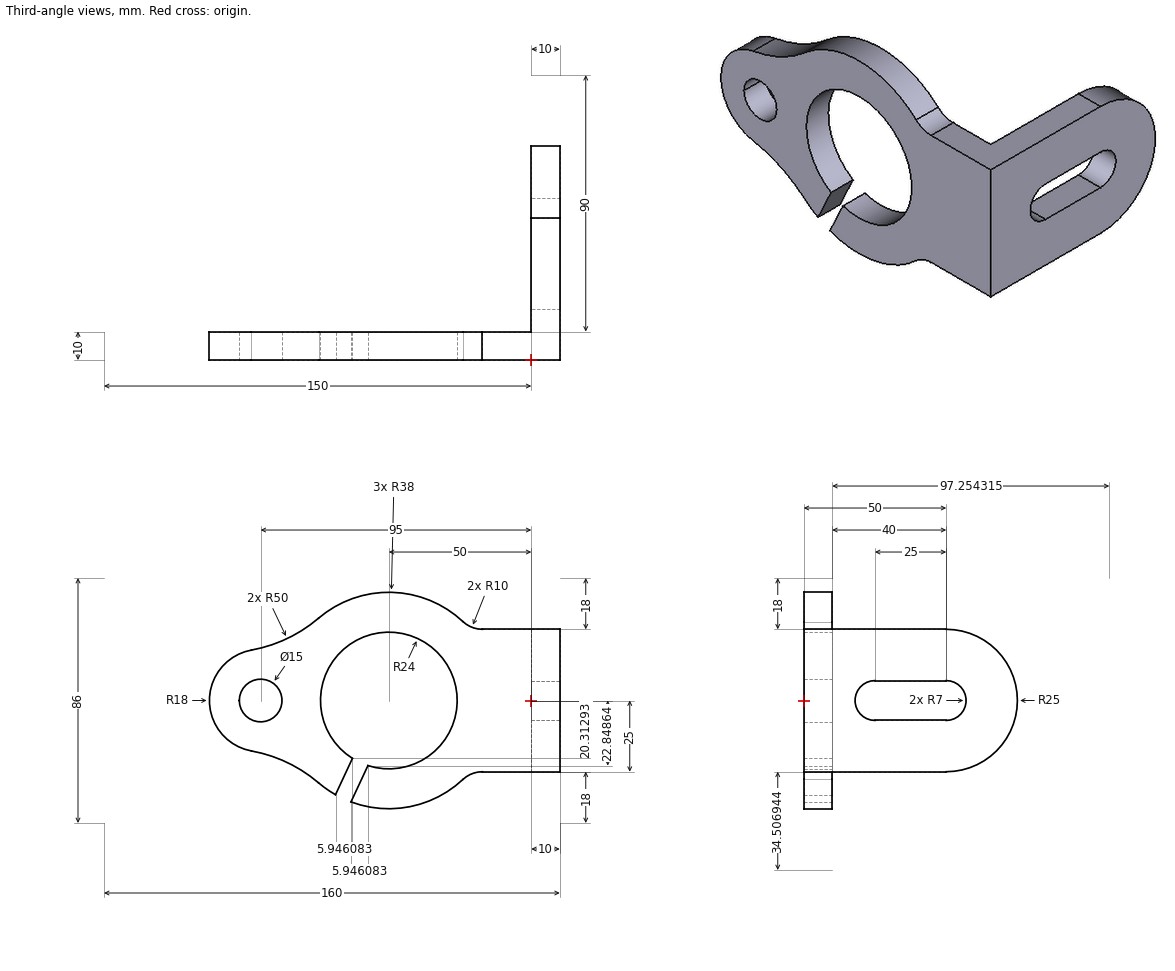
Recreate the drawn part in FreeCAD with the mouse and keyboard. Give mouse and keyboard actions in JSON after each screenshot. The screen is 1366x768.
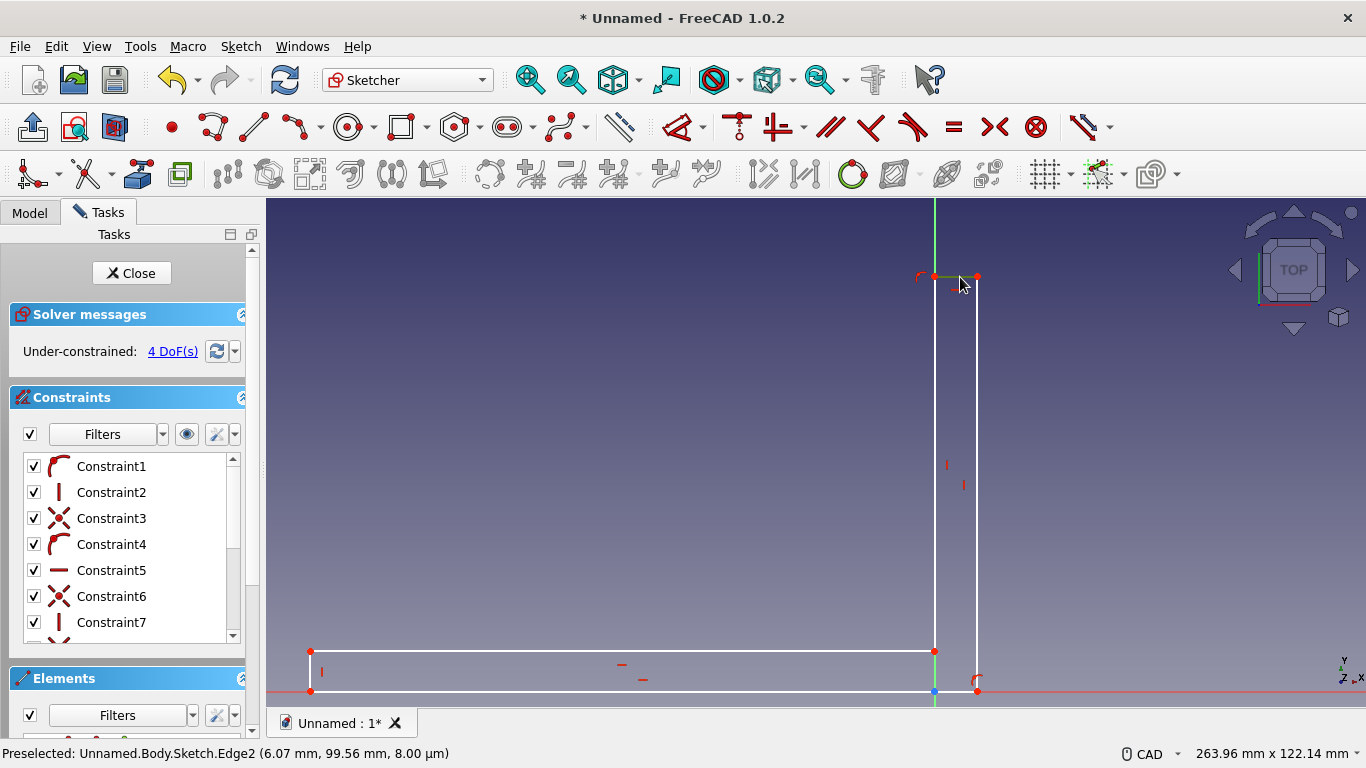
{"action": "key", "text": "l"}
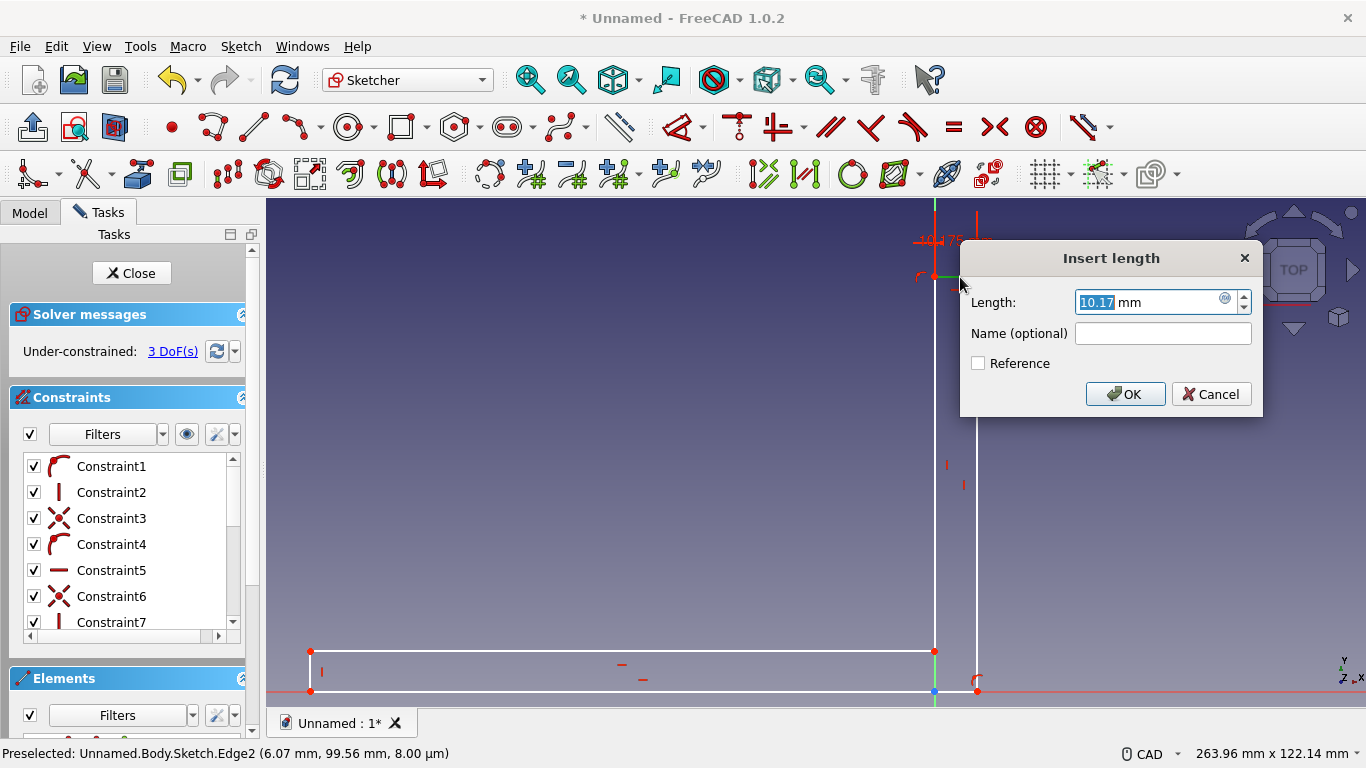
{"action": "type", "text": "10"}
{"action": "key", "text": "Return"}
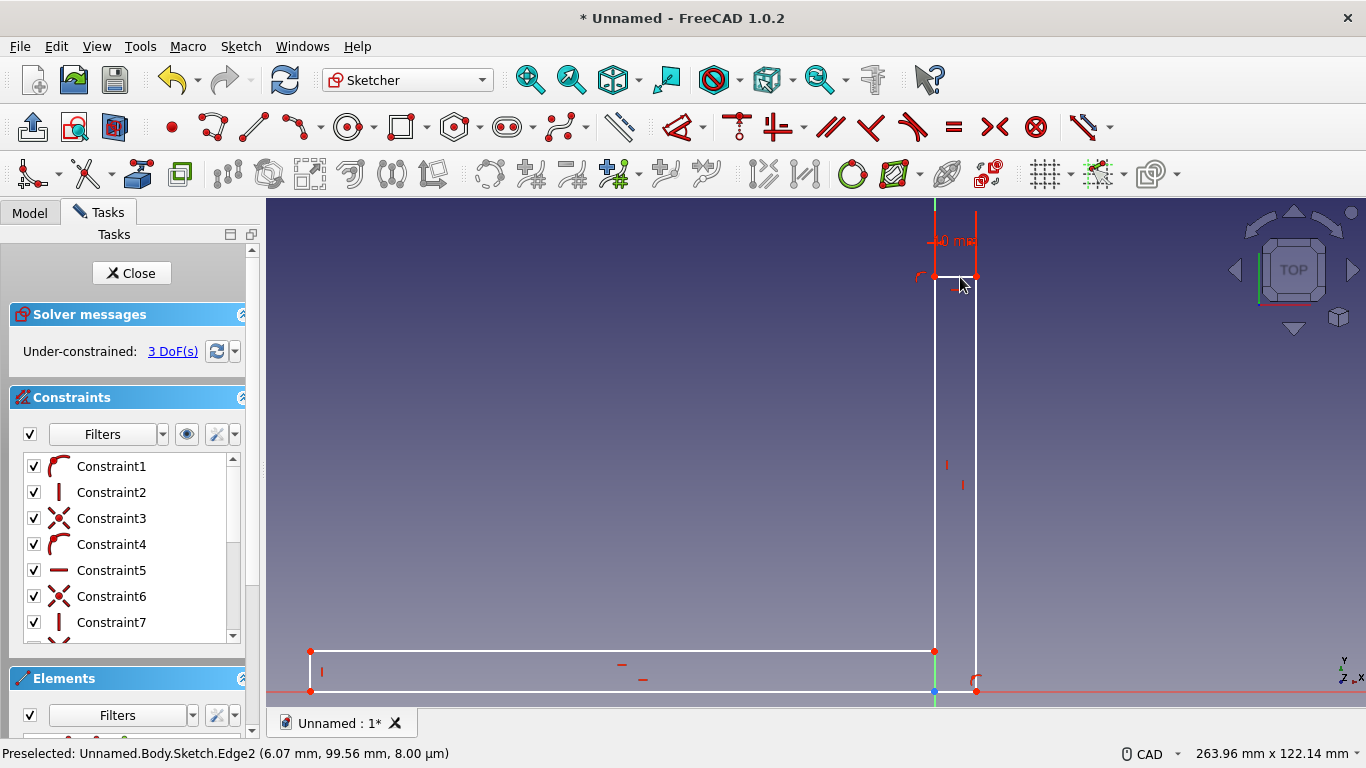
{"action": "left_click", "coordinate": [935, 389]}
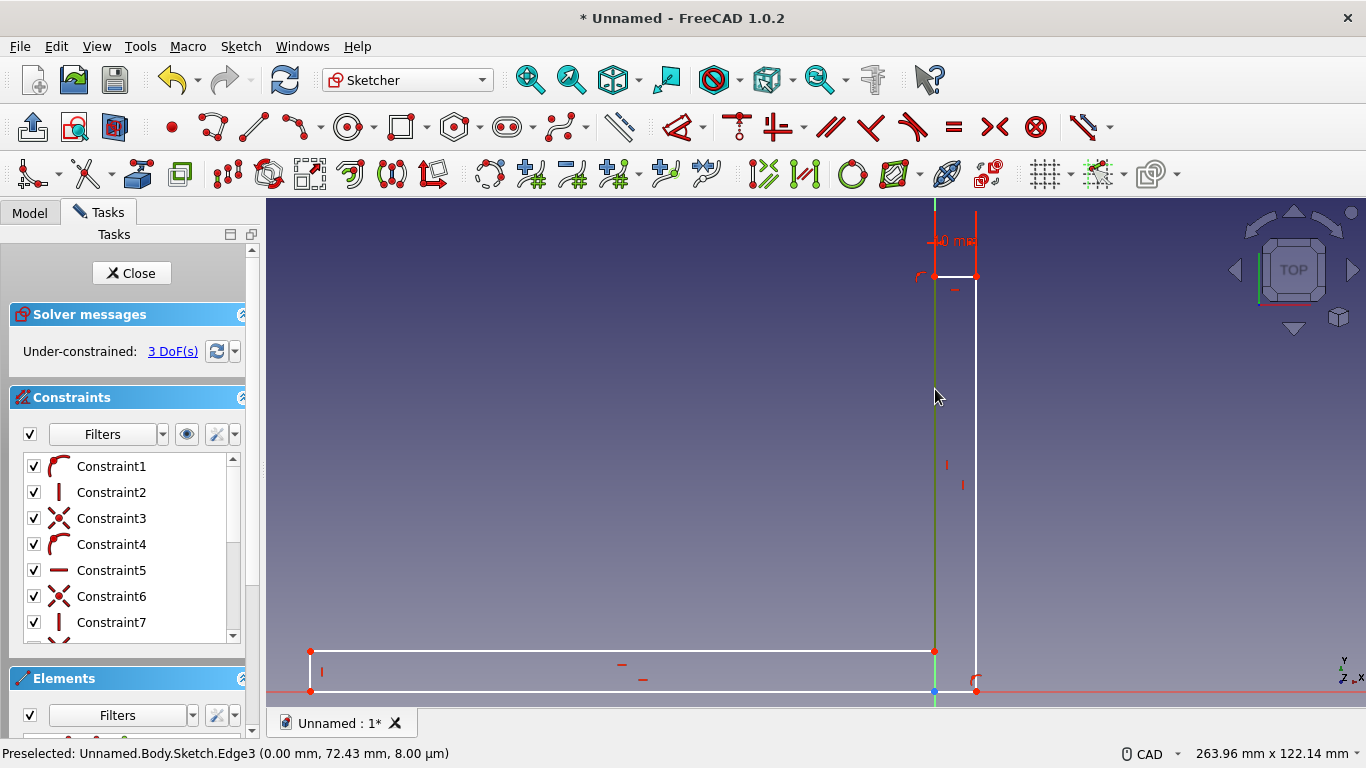
{"action": "key", "text": "i"}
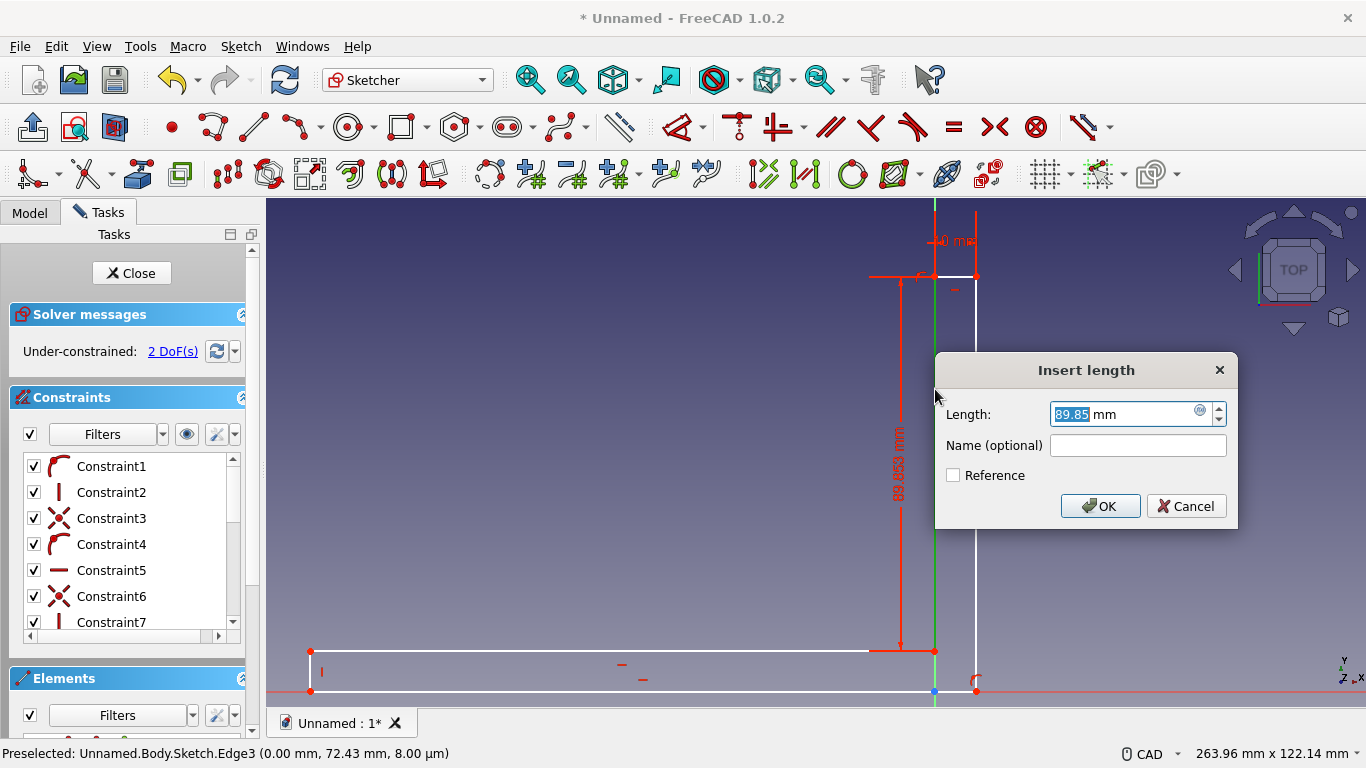
{"action": "type", "text": "90"}
{"action": "key", "text": "Return"}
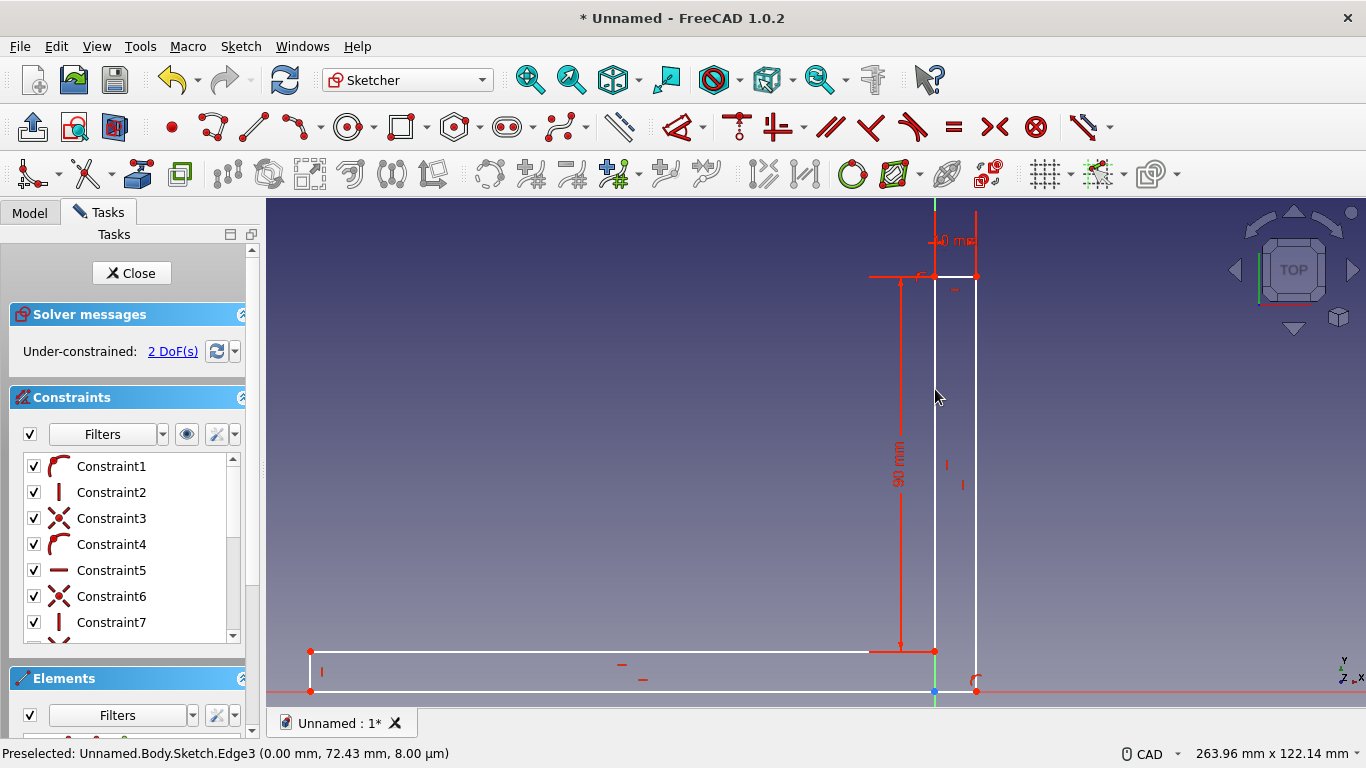
{"action": "left_click", "coordinate": [310, 664]}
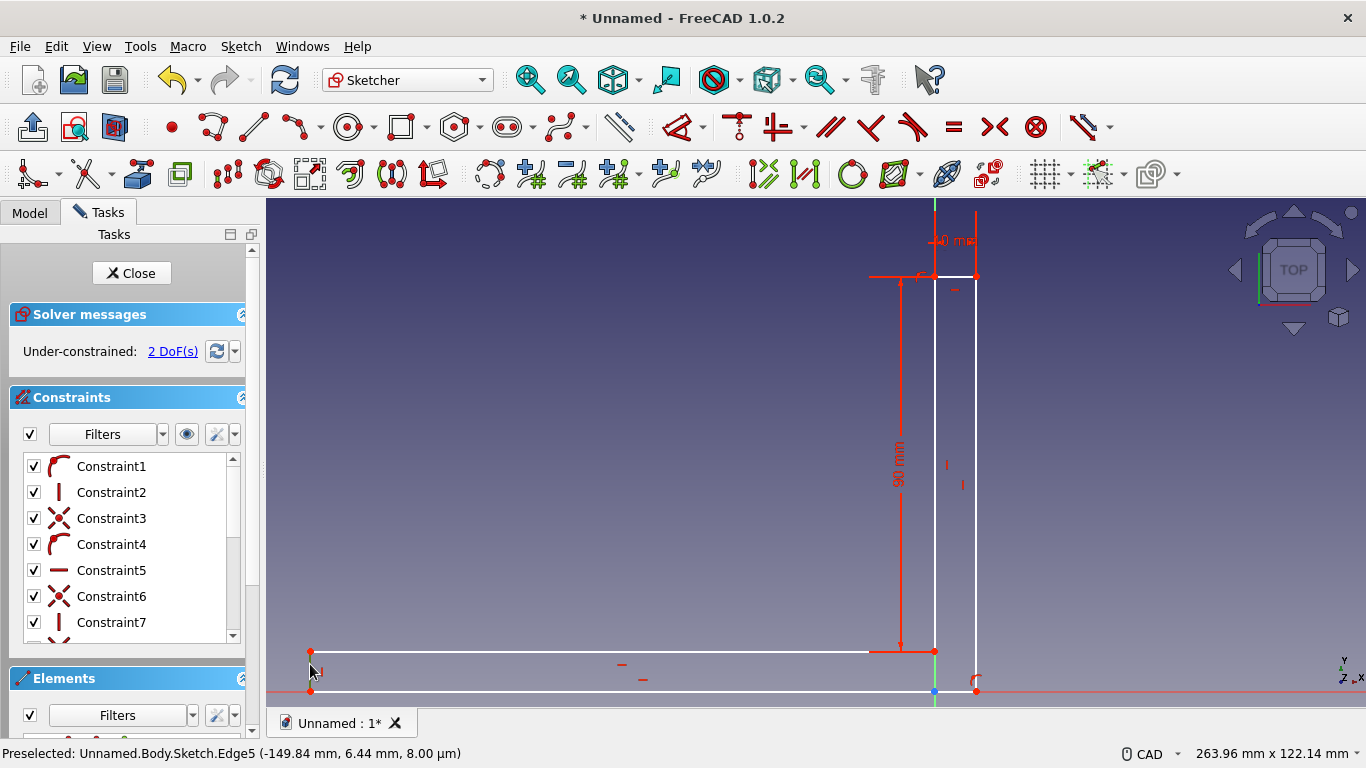
{"action": "key", "text": "i"}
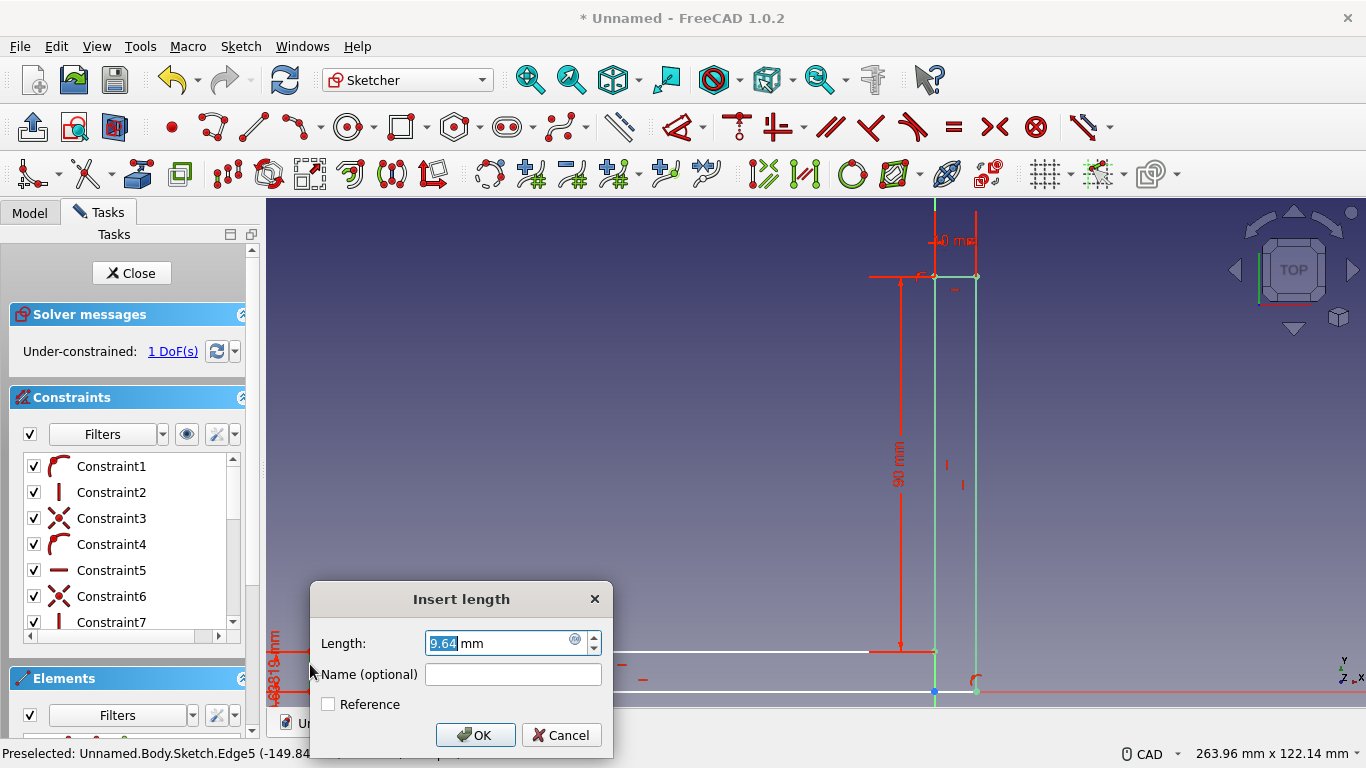
{"action": "type", "text": "10"}
{"action": "key", "text": "Return"}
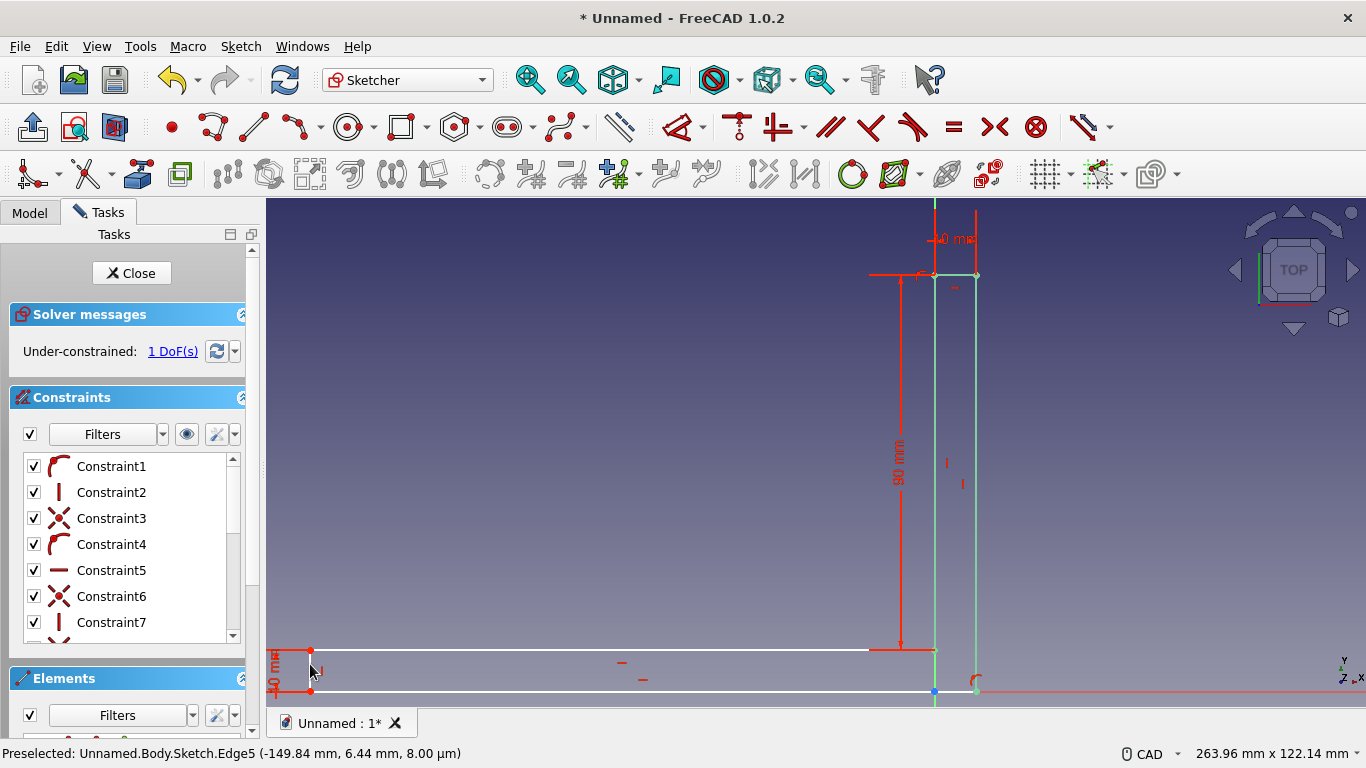
{"action": "left_click", "coordinate": [747, 650]}